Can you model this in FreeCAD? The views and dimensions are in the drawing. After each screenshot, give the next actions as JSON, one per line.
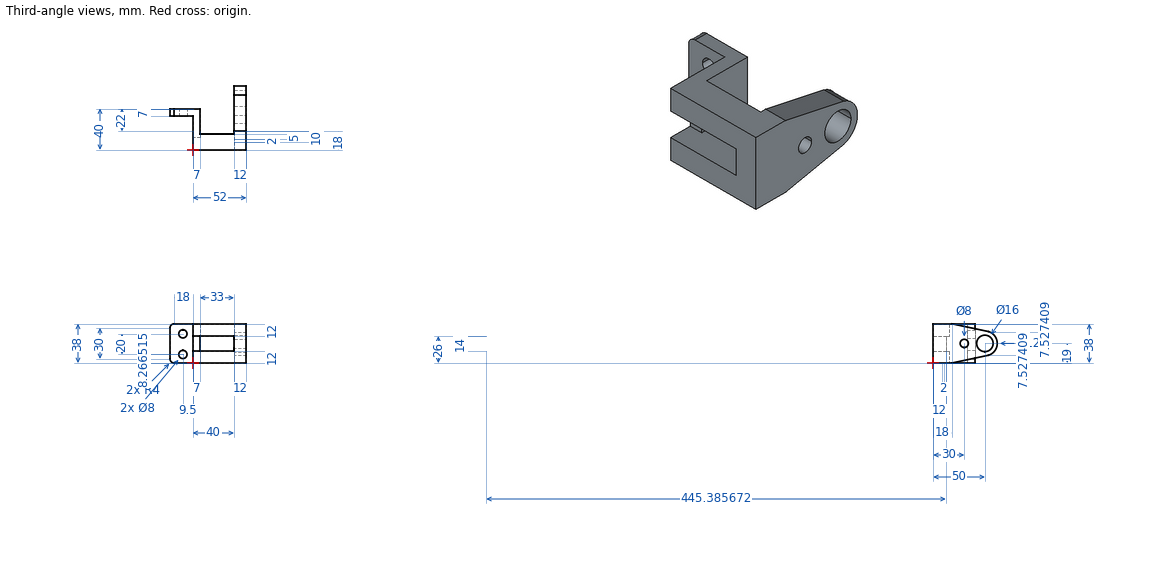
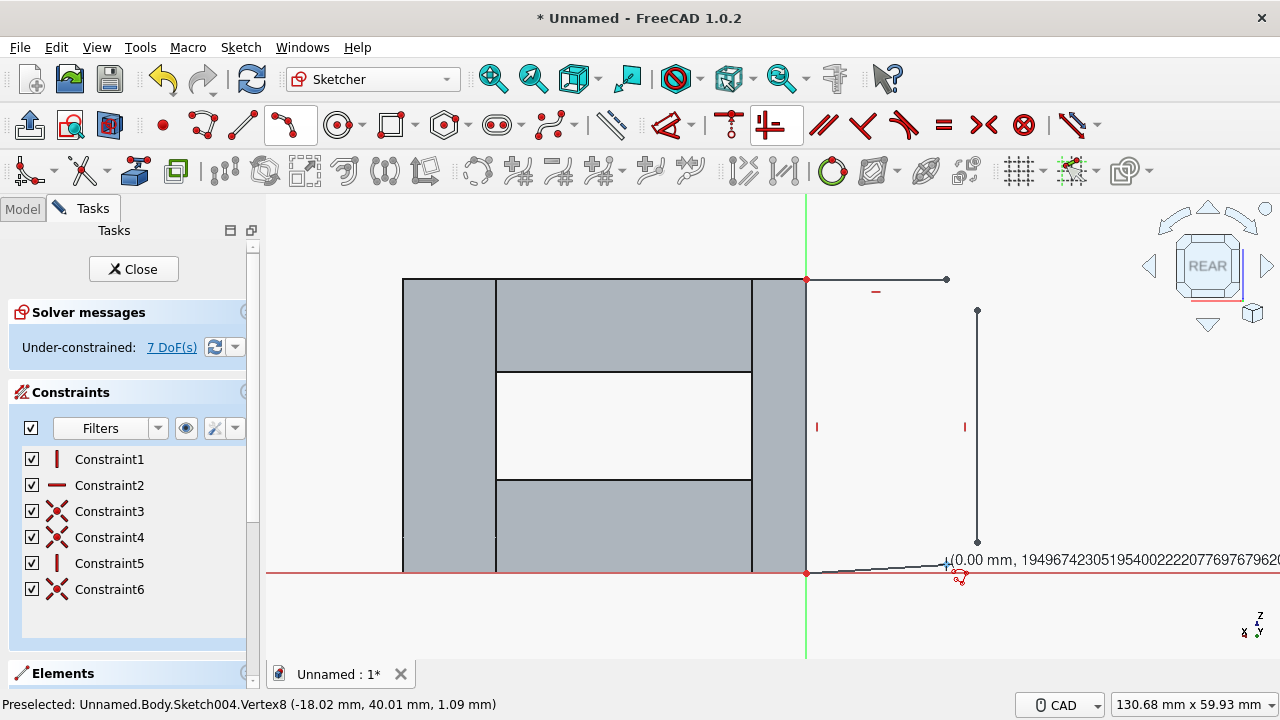
{"action": "left_click", "coordinate": [284, 126]}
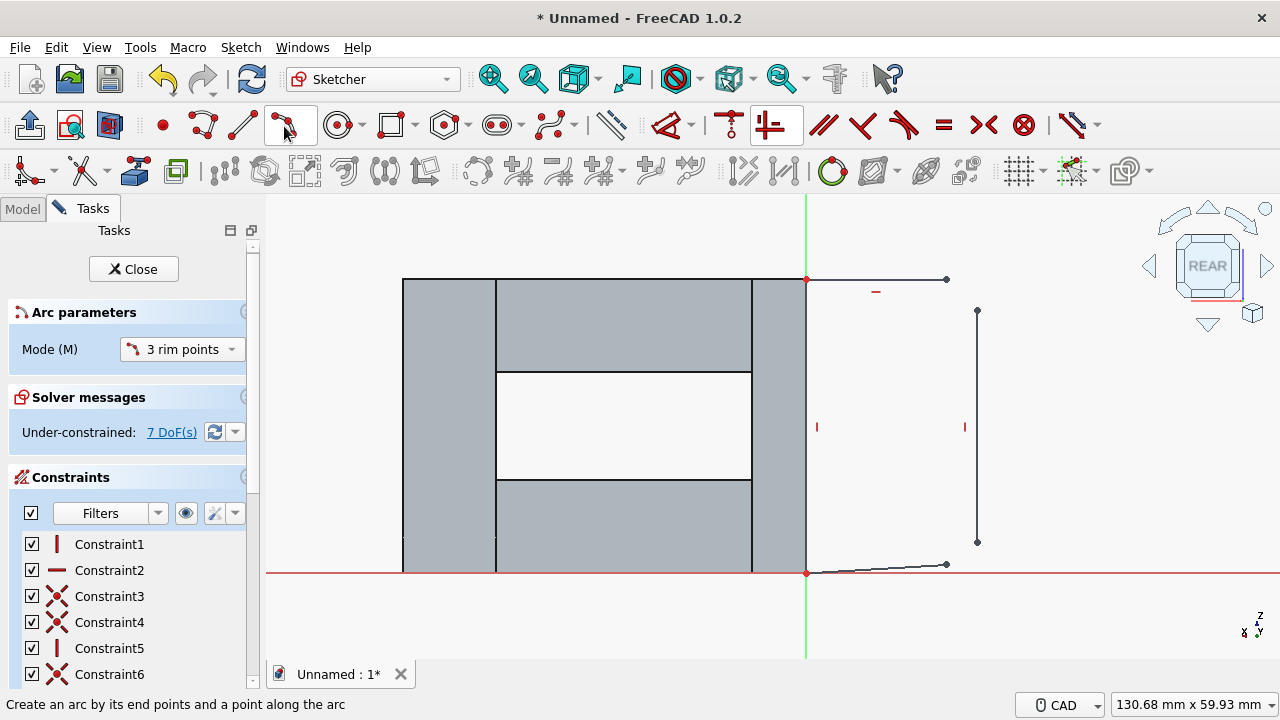
{"action": "left_click", "coordinate": [977, 311]}
{"action": "left_click", "coordinate": [946, 280]}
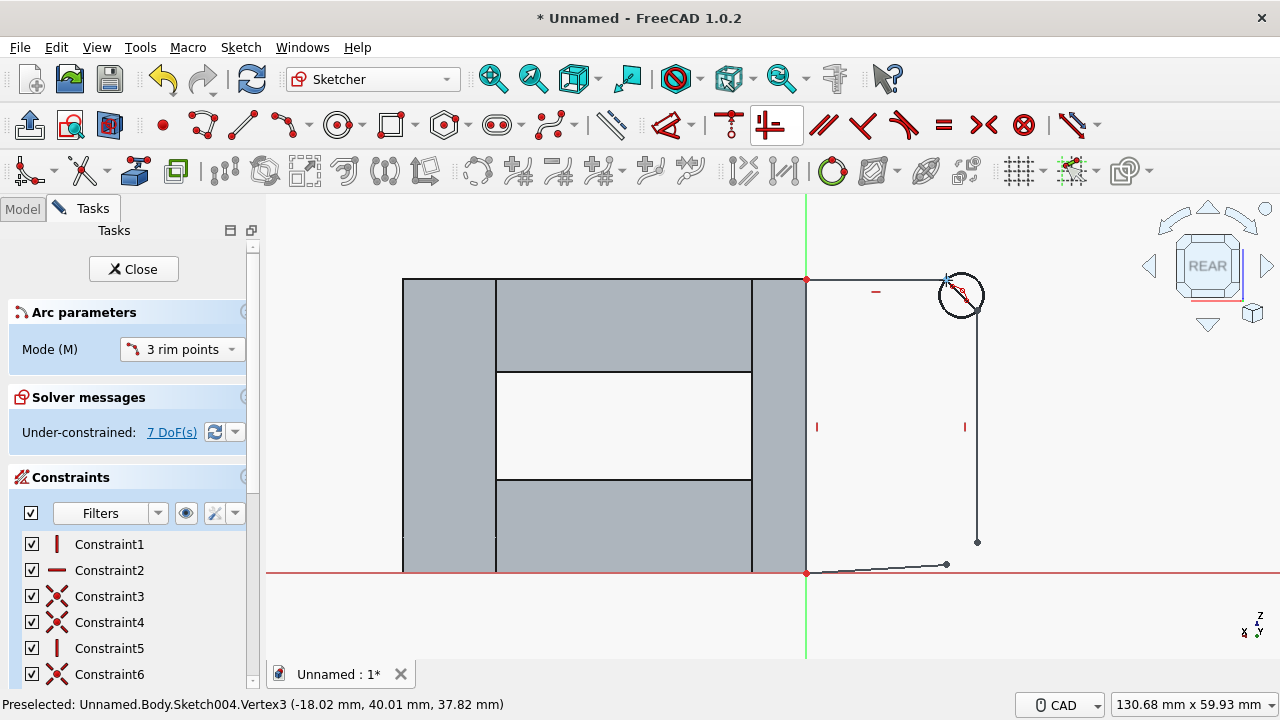
{"action": "scroll", "coordinate": [968, 288], "scroll_direction": "up", "scroll_amount": 3}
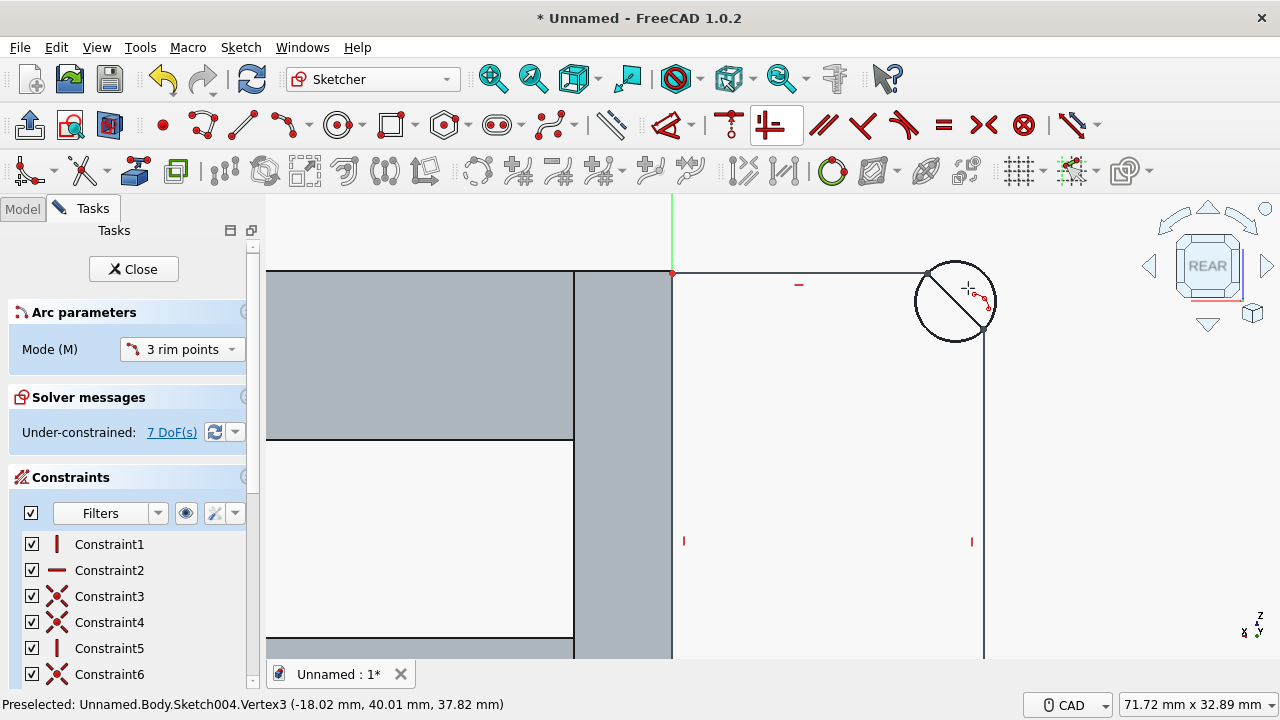
{"action": "left_click", "coordinate": [967, 287]}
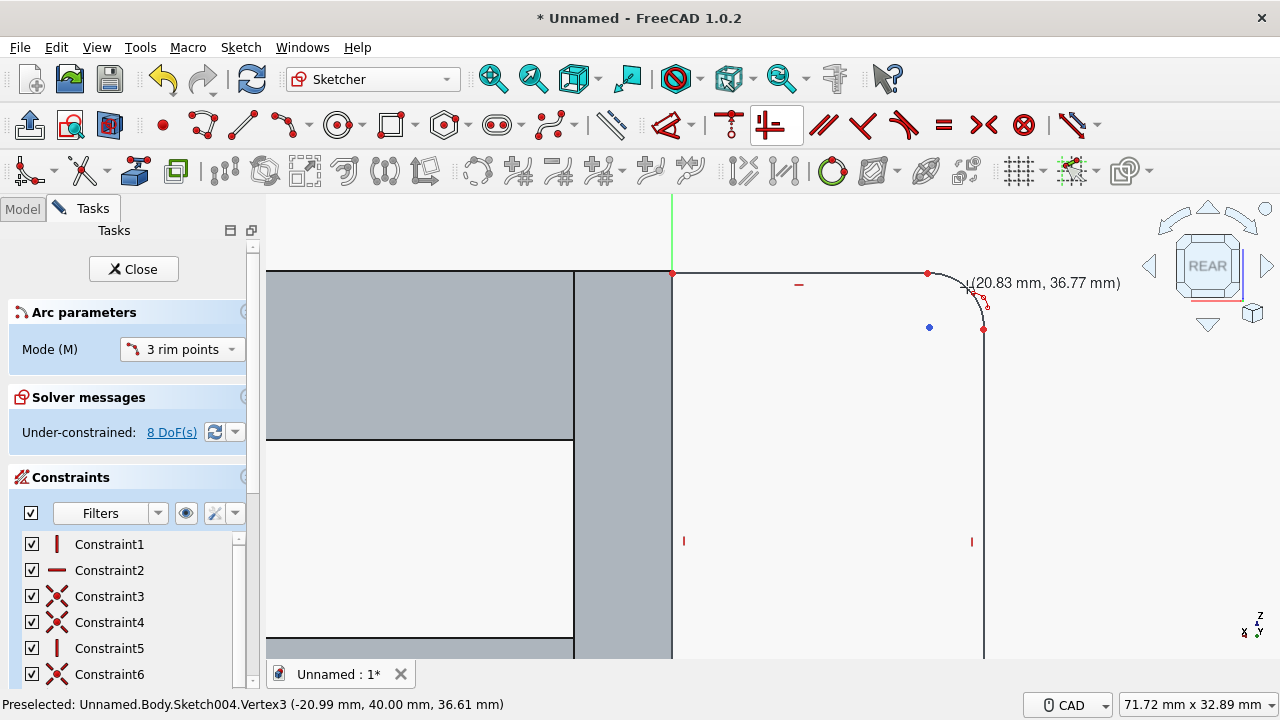
{"action": "scroll", "coordinate": [554, 289], "scroll_direction": "down", "scroll_amount": 3}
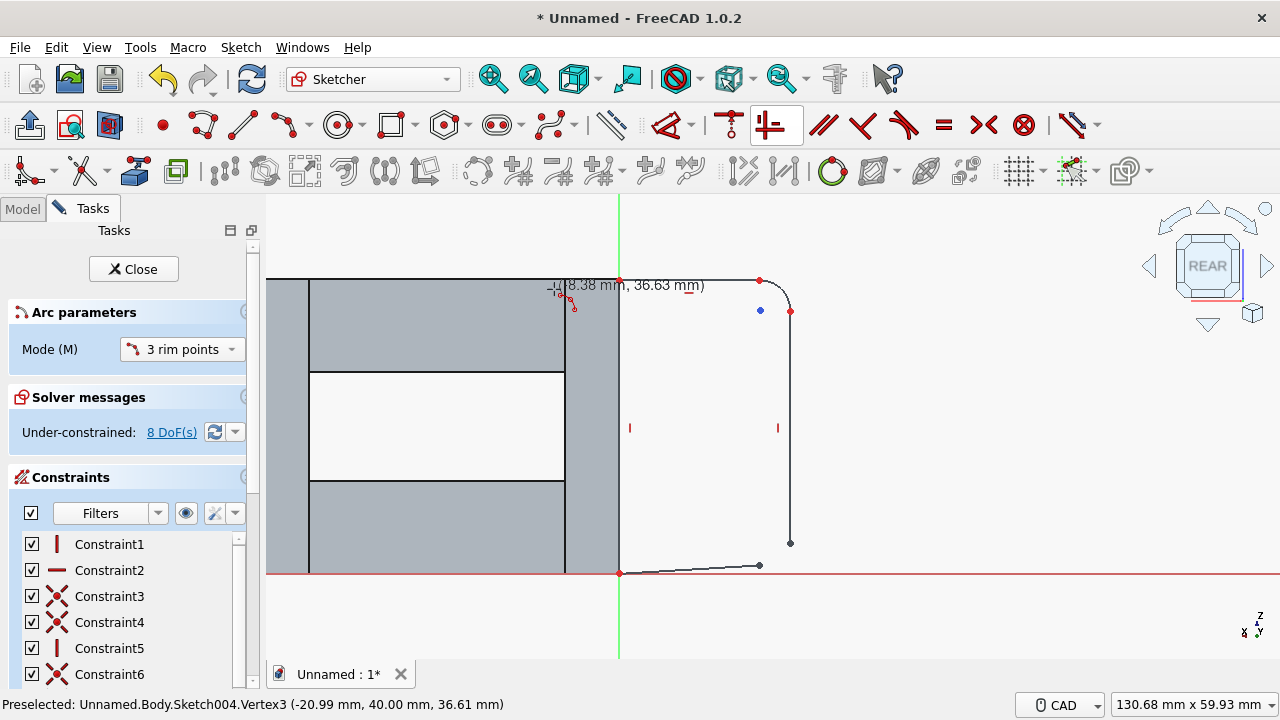
{"action": "left_click", "coordinate": [759, 565]}
{"action": "left_click", "coordinate": [790, 543]}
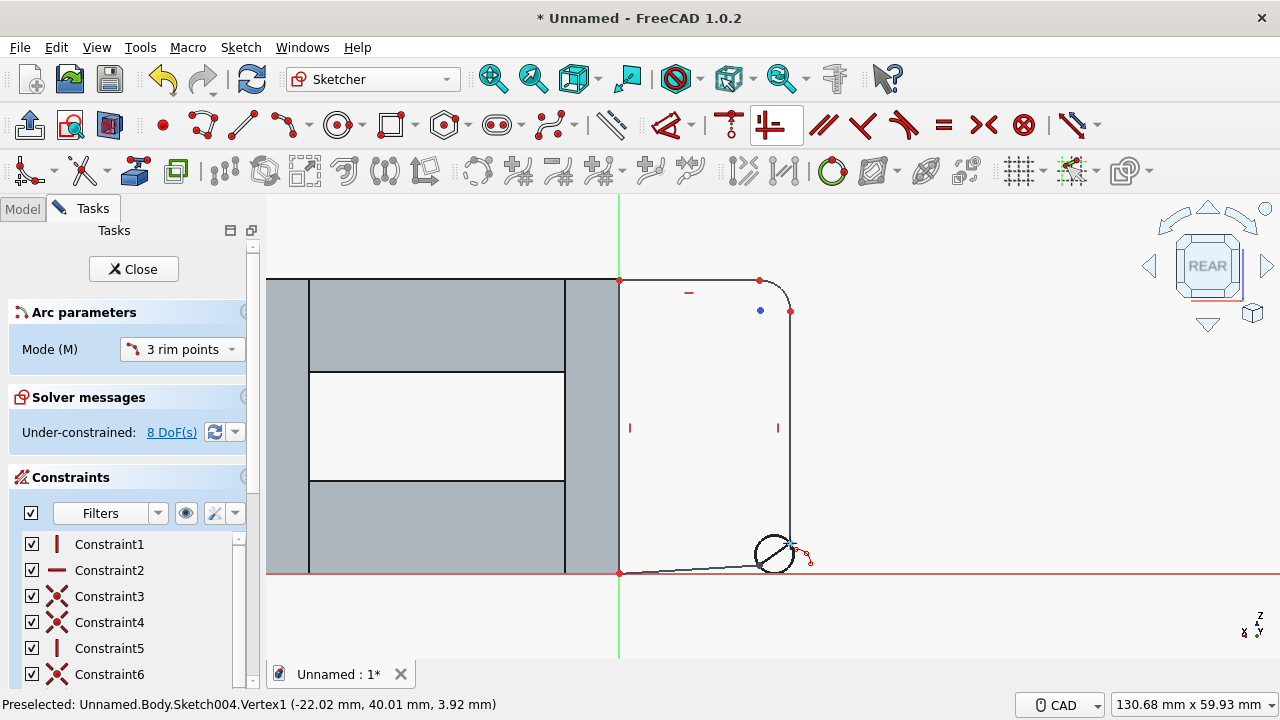
{"action": "scroll", "coordinate": [781, 565], "scroll_direction": "up", "scroll_amount": 3}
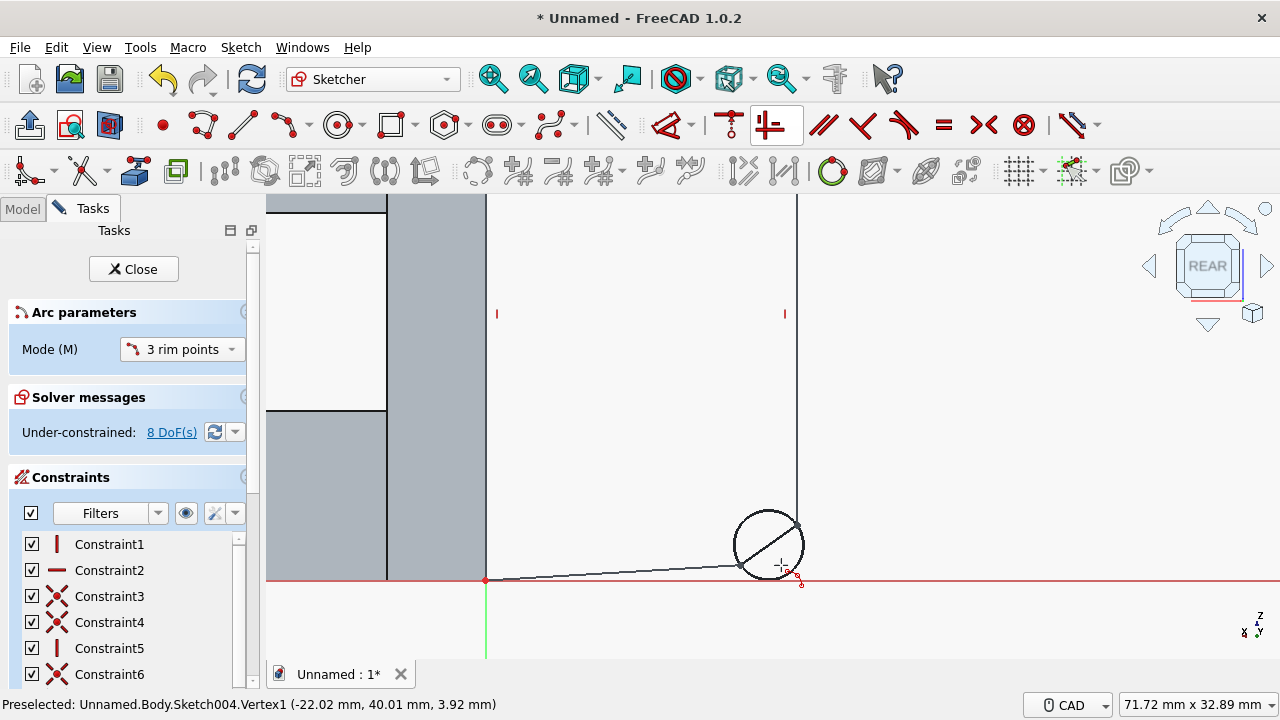
{"action": "left_click", "coordinate": [780, 564]}
{"action": "key", "text": "Escape"}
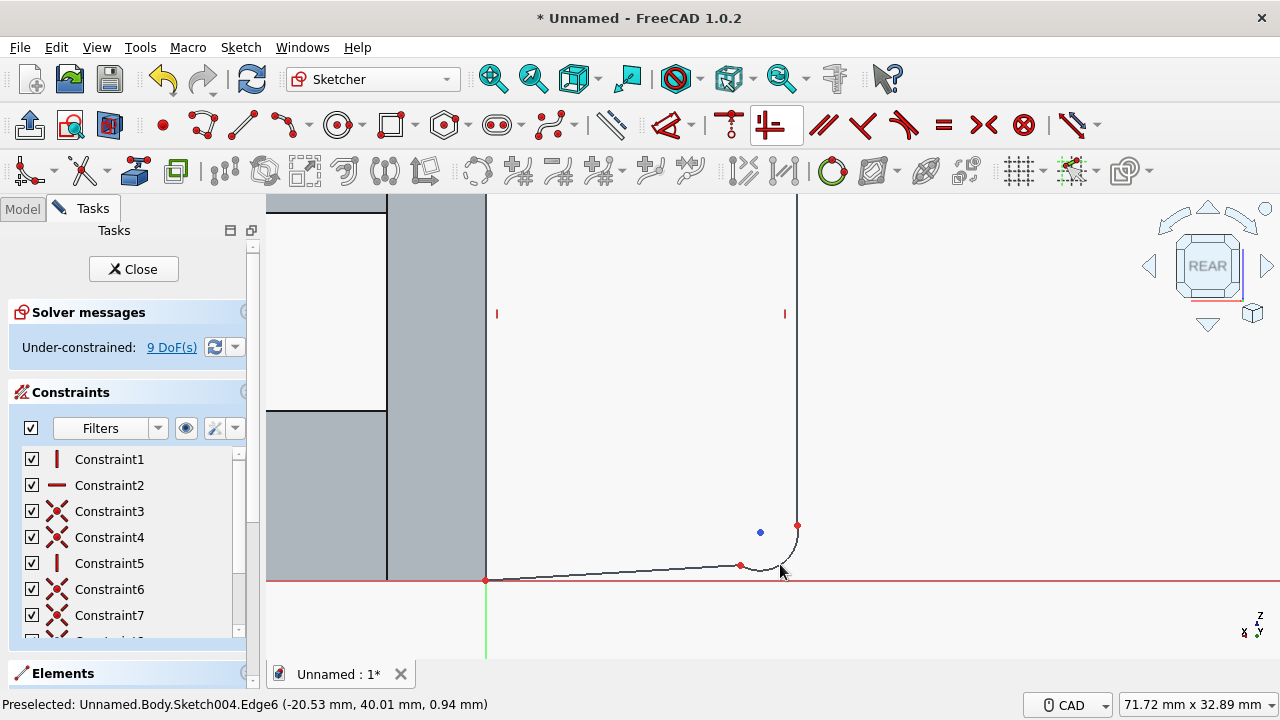
{"action": "left_click", "coordinate": [797, 398]}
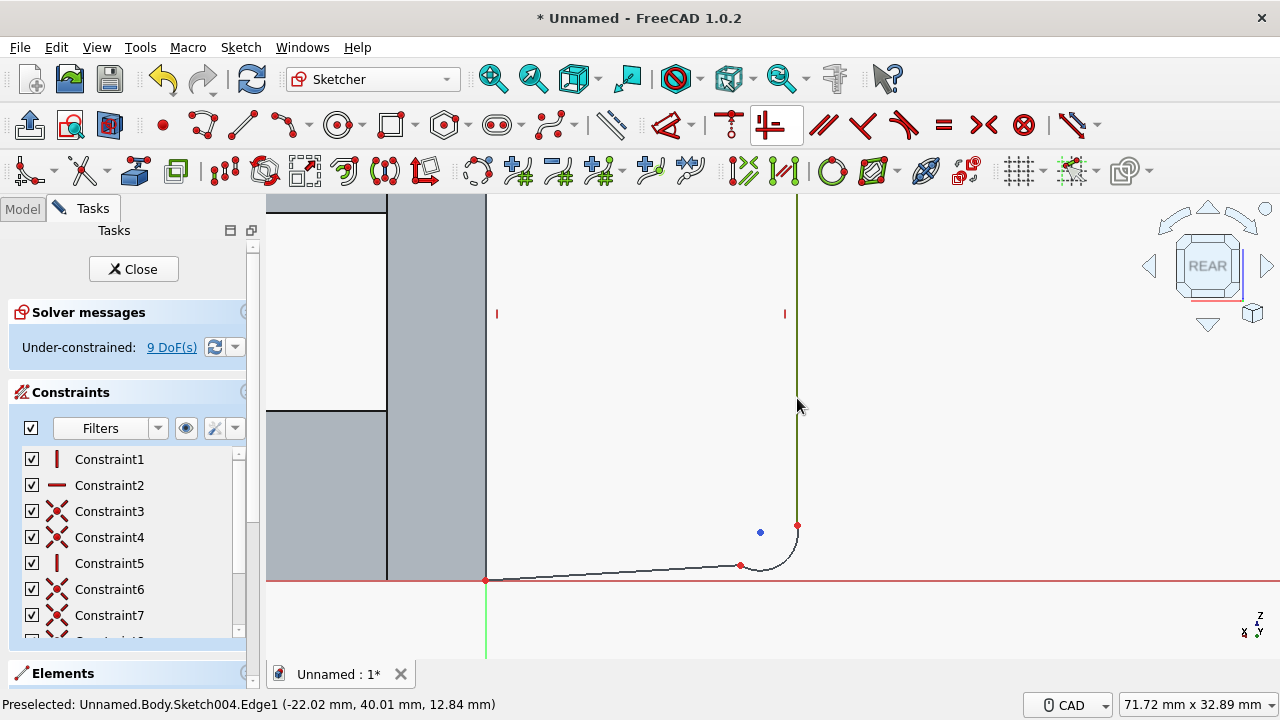
{"action": "scroll", "coordinate": [781, 566], "scroll_direction": "down", "scroll_amount": 3}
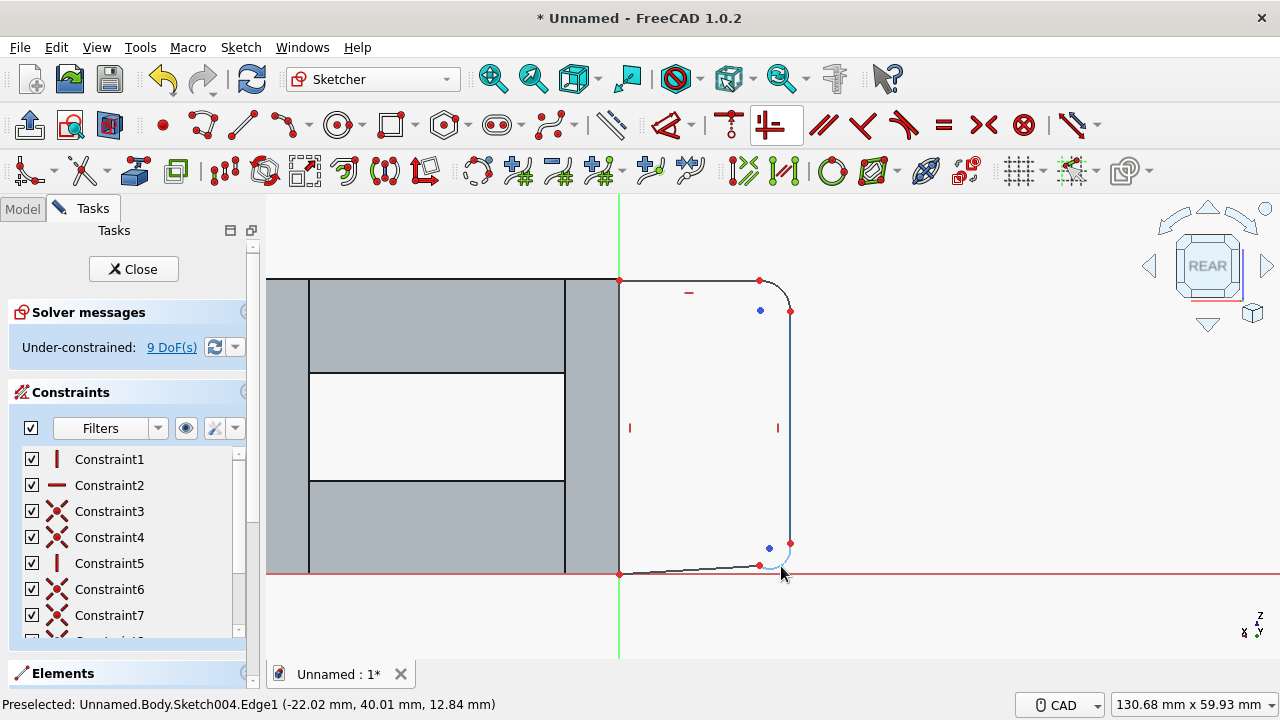
{"action": "left_click", "coordinate": [787, 298]}